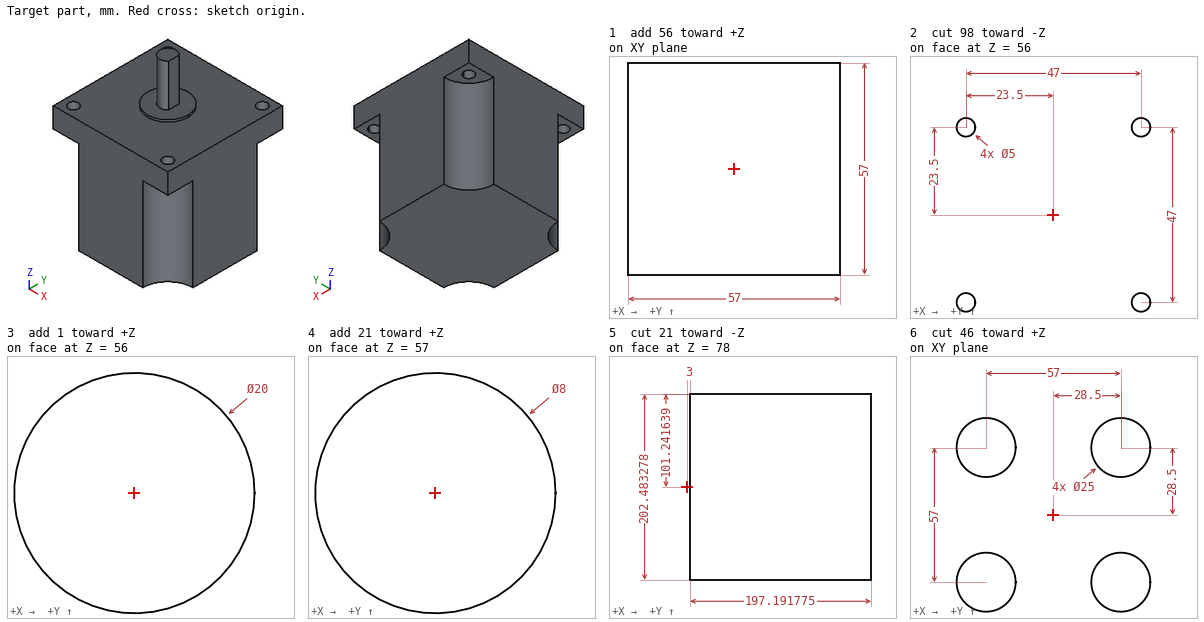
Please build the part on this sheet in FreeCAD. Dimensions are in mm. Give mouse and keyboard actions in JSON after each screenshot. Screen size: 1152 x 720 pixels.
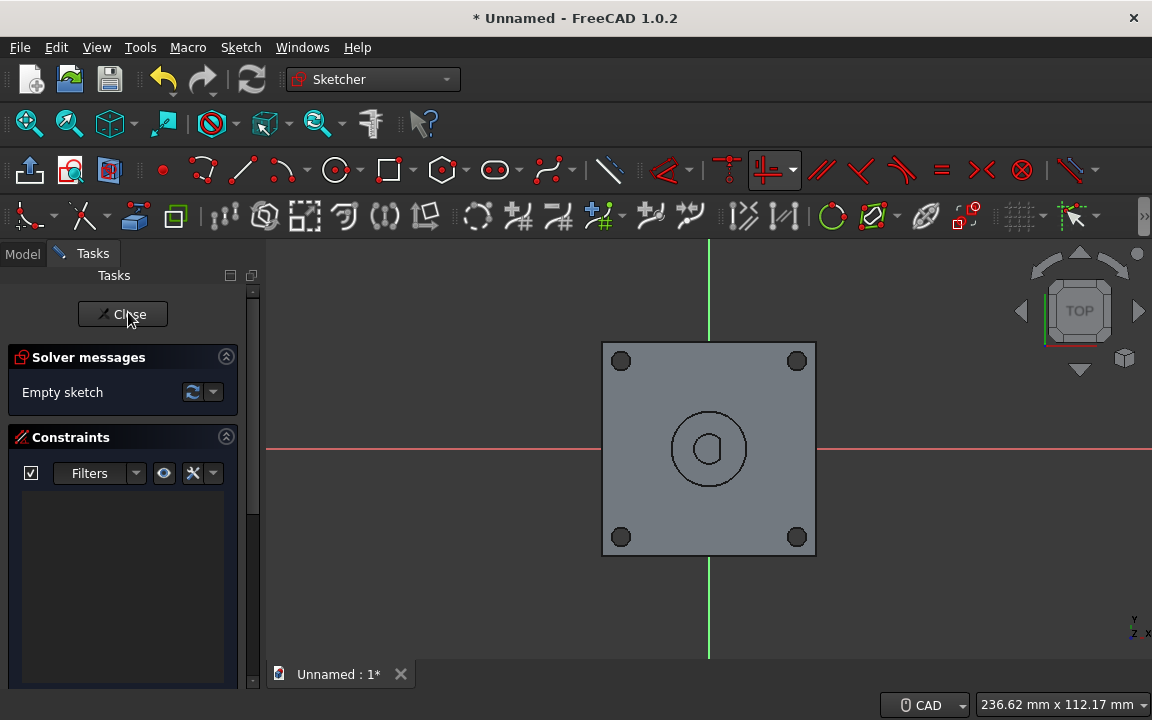
{"action": "left_click", "coordinate": [110, 170]}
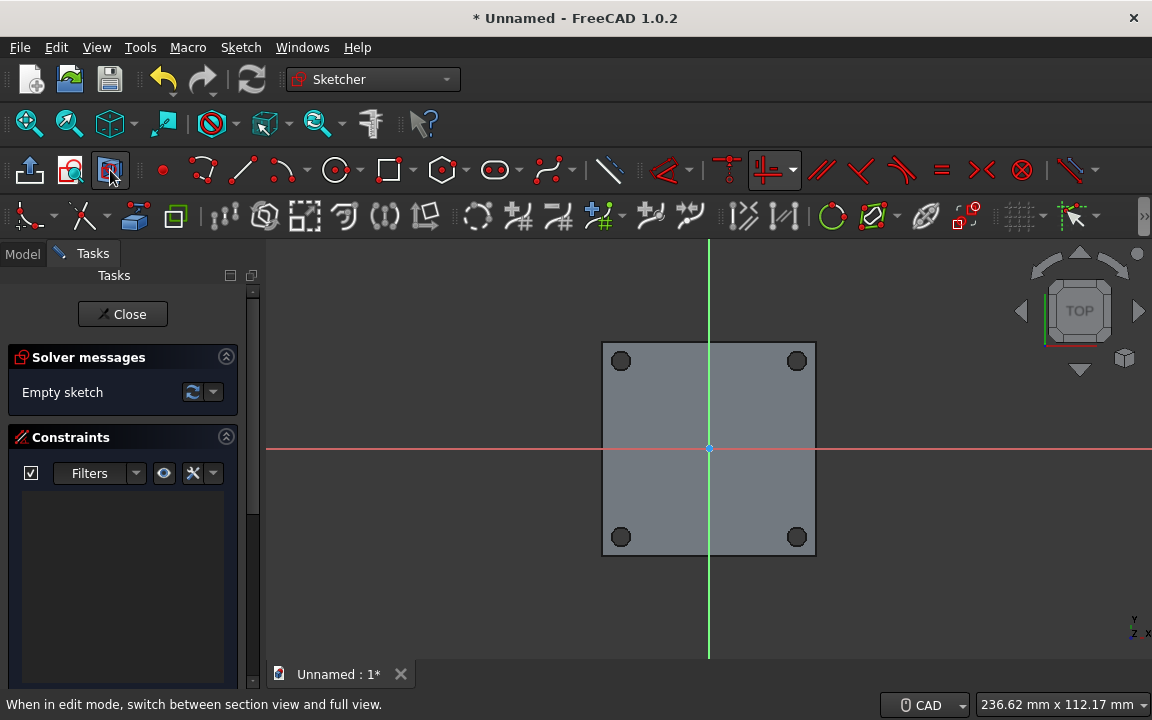
{"action": "left_click", "coordinate": [336, 170]}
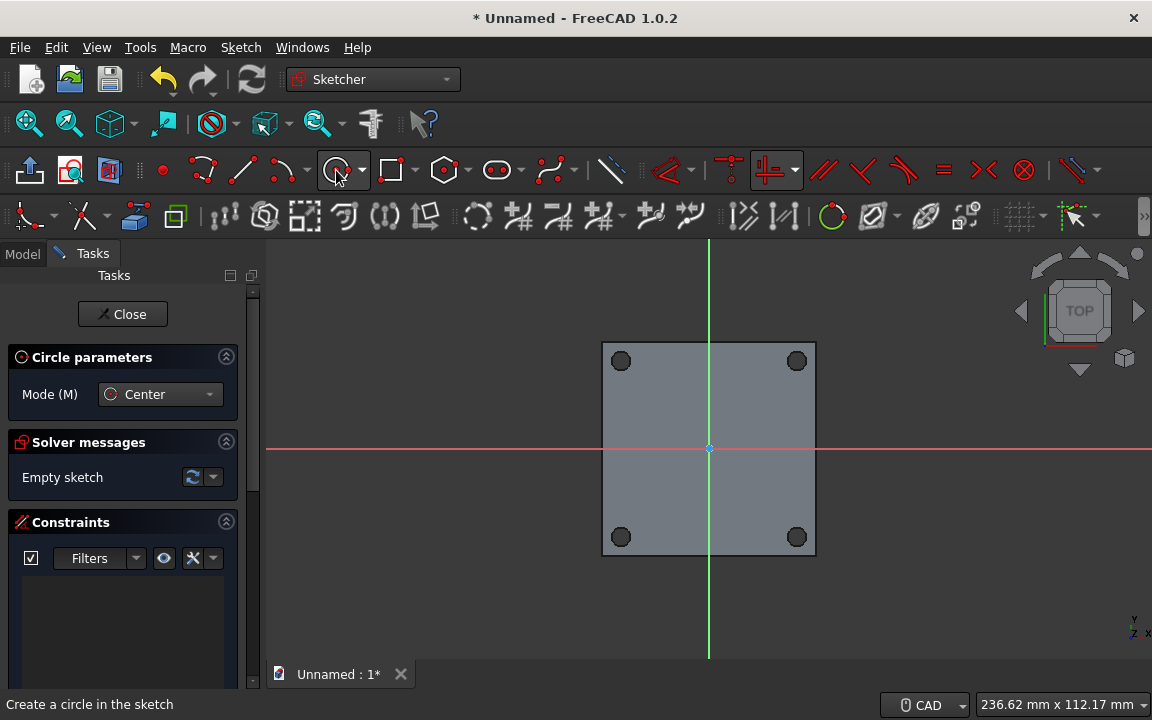
{"action": "left_click", "coordinate": [816, 342]}
{"action": "left_click", "coordinate": [849, 309]}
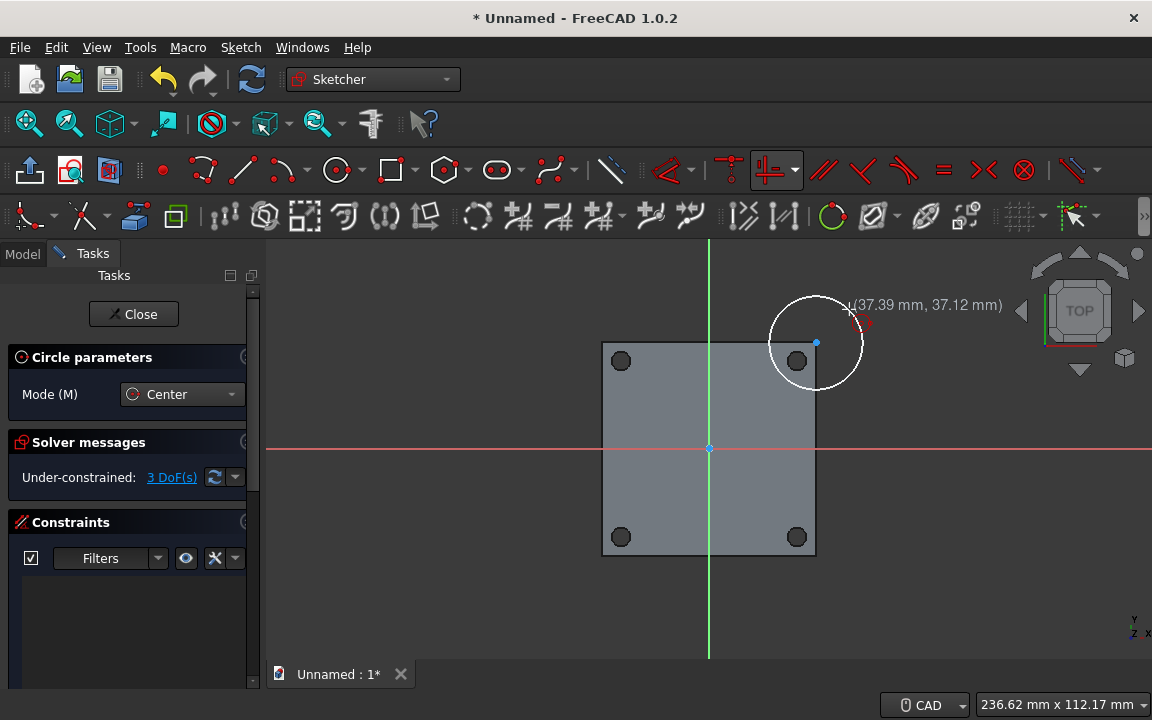
{"action": "left_click", "coordinate": [602, 342]}
{"action": "left_click", "coordinate": [635, 309]}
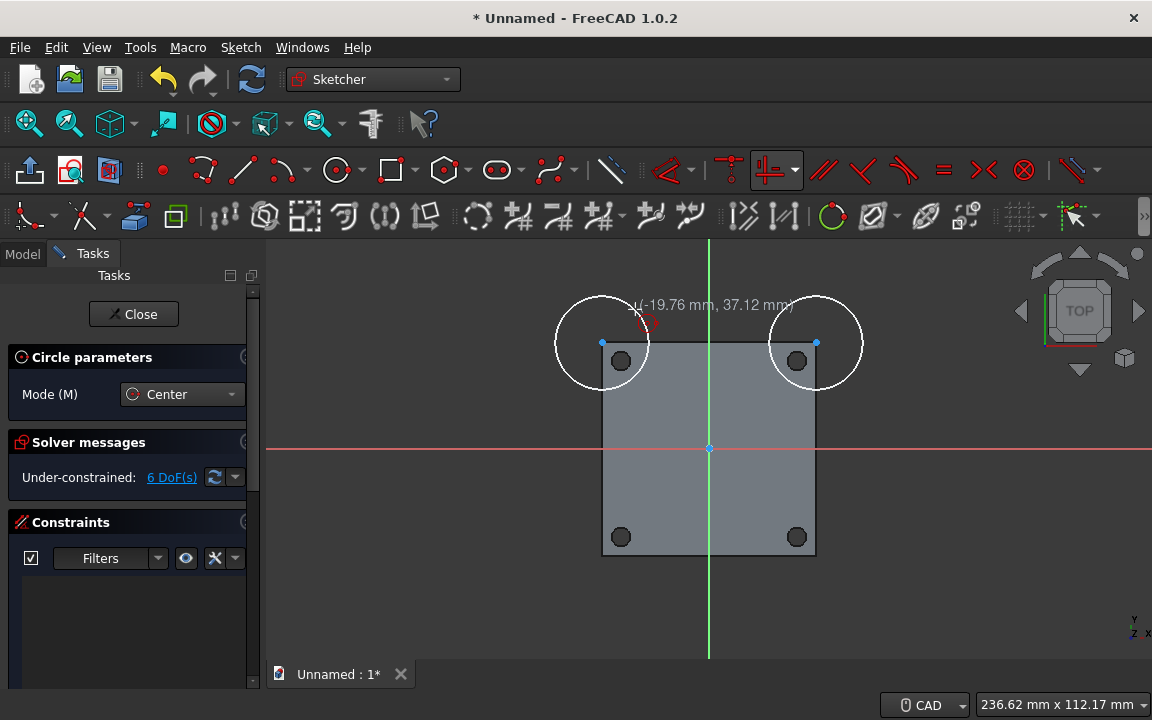
{"action": "left_click", "coordinate": [602, 556]}
{"action": "left_click", "coordinate": [635, 523]}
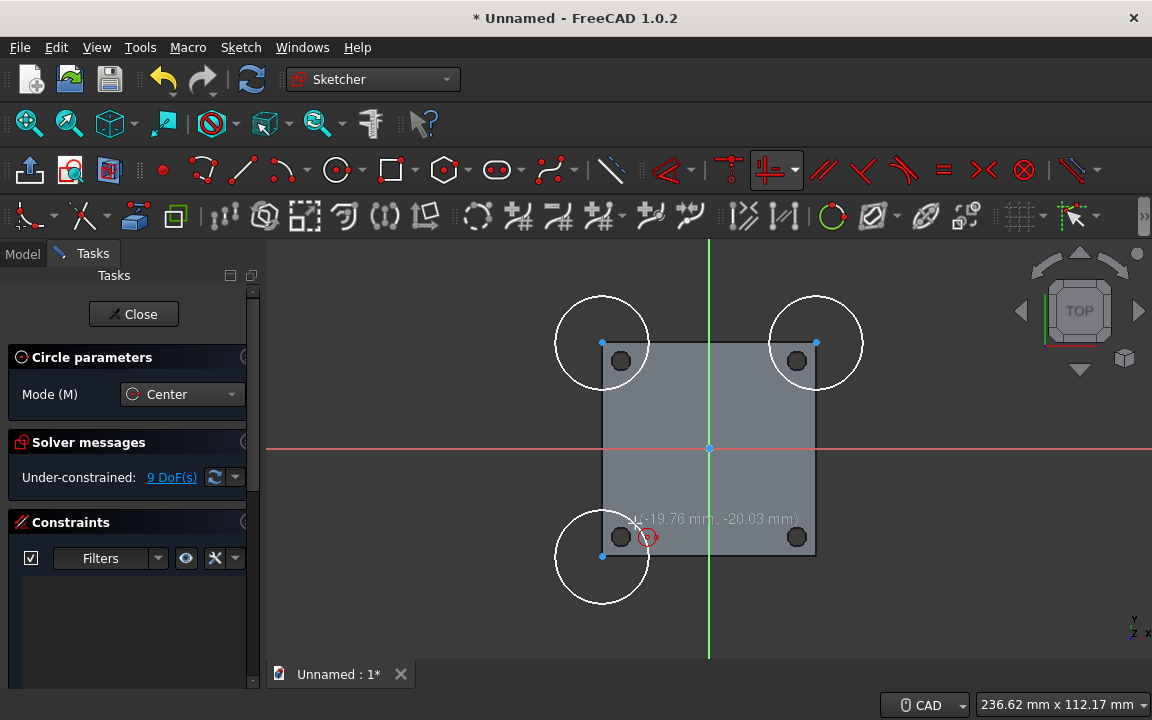
{"action": "left_click", "coordinate": [816, 556]}
{"action": "left_click", "coordinate": [849, 523]}
{"action": "key", "text": "Escape"}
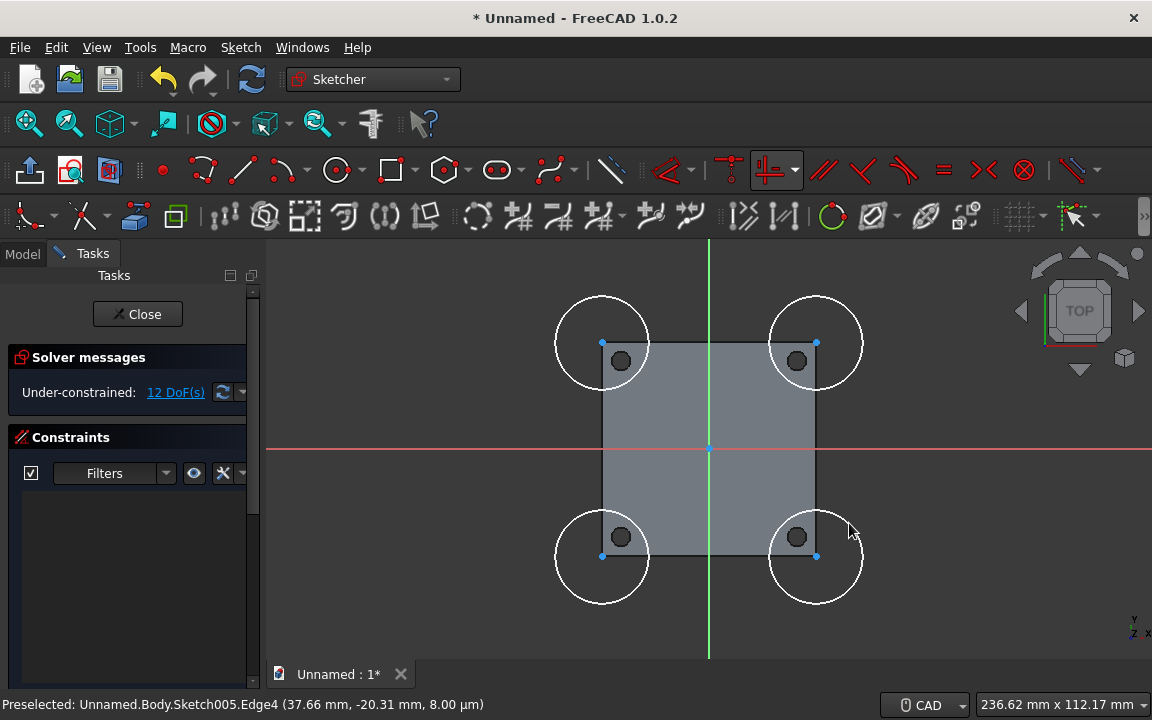
{"action": "left_click", "coordinate": [849, 310]}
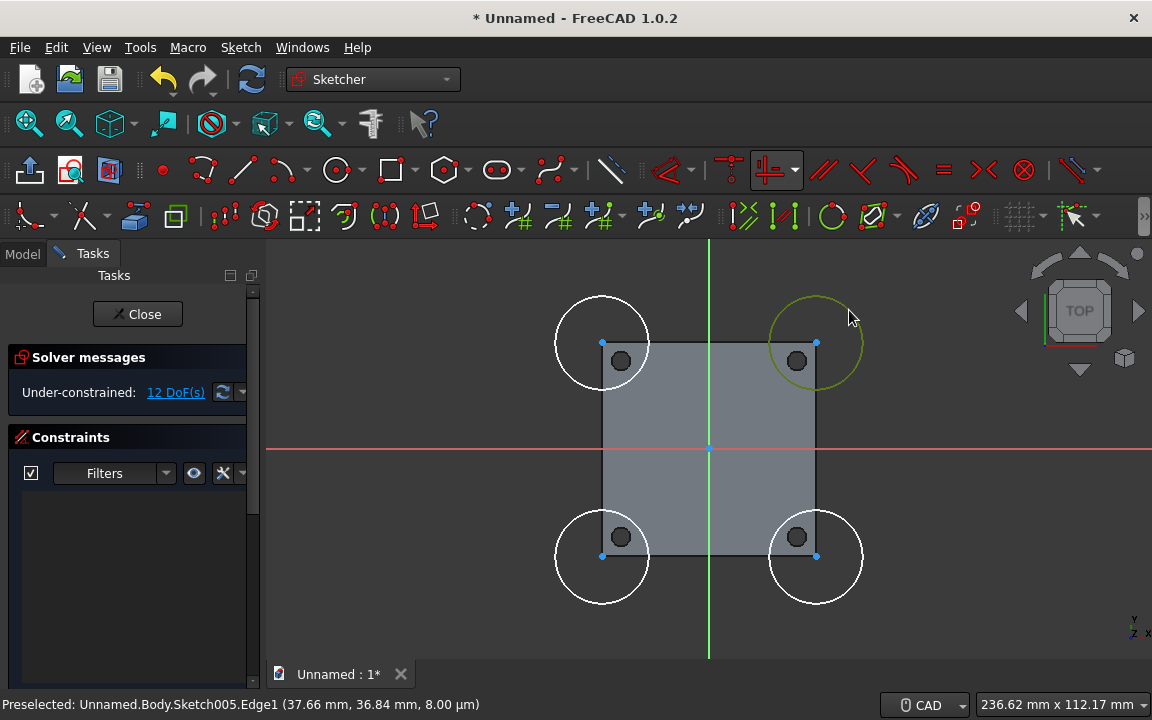
{"action": "left_click", "coordinate": [635, 310]}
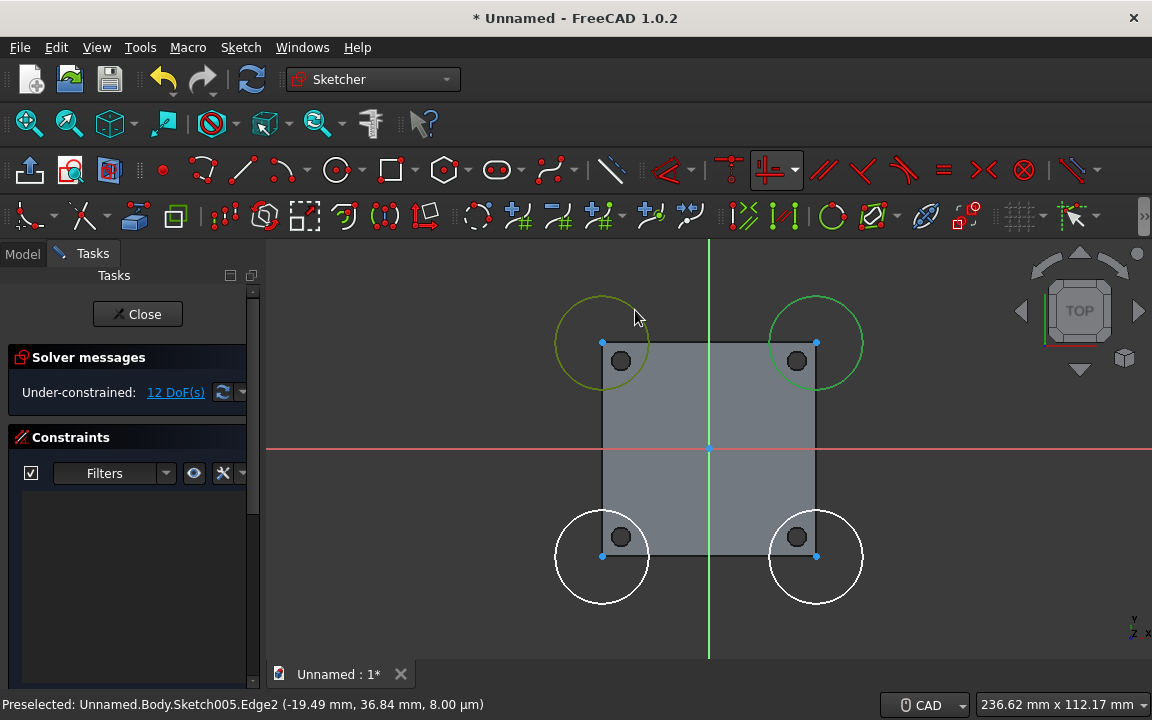
{"action": "left_click", "coordinate": [635, 524]}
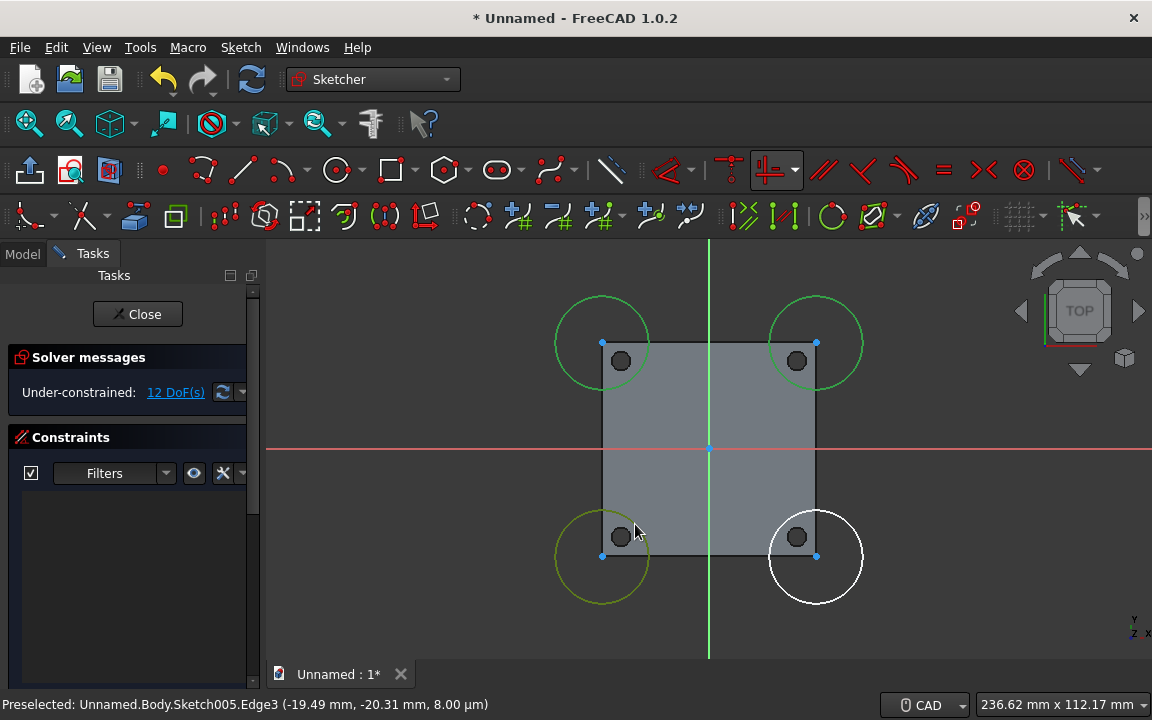
{"action": "left_click", "coordinate": [849, 524]}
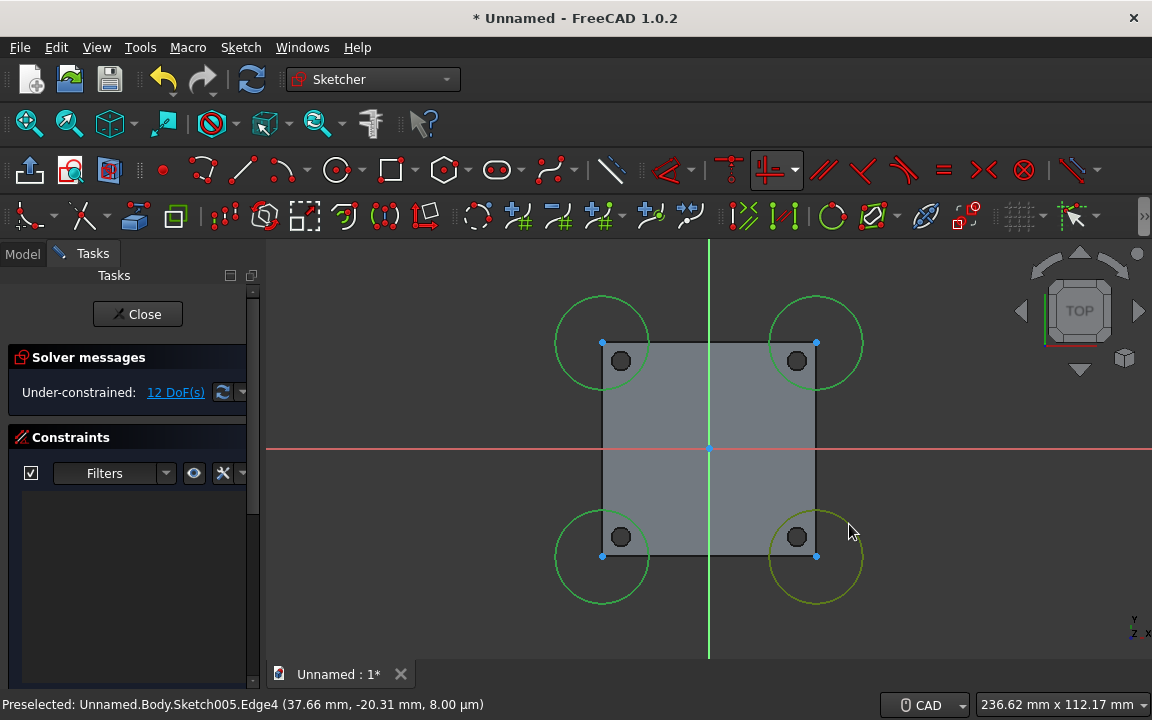
{"action": "left_click", "coordinate": [944, 170]}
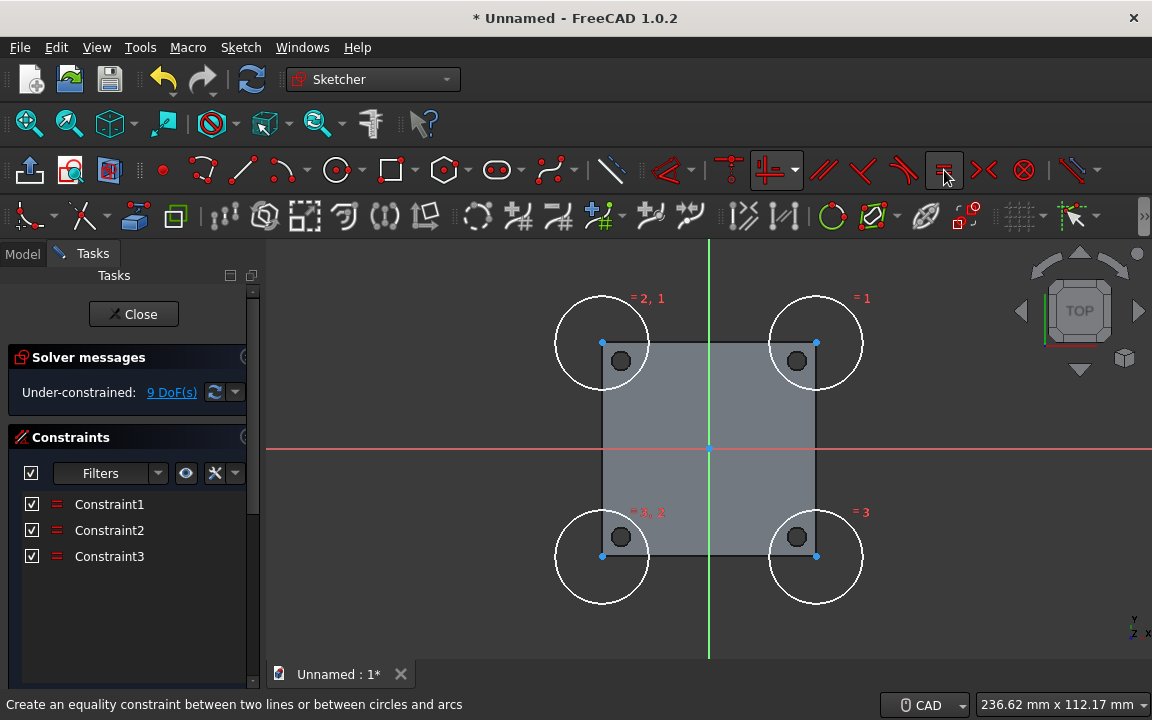
{"action": "left_click", "coordinate": [816, 343]}